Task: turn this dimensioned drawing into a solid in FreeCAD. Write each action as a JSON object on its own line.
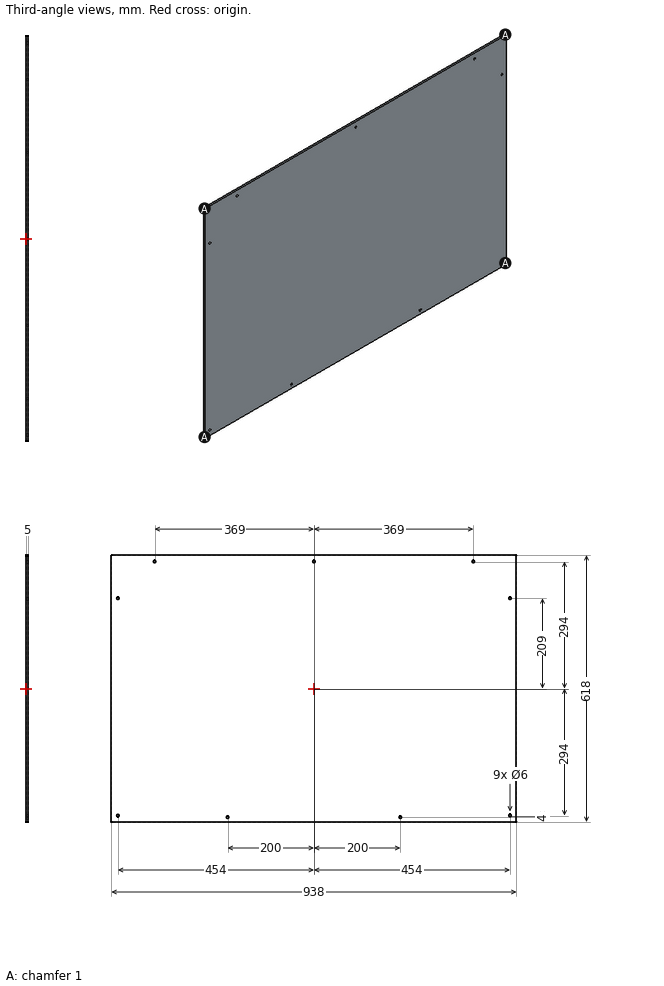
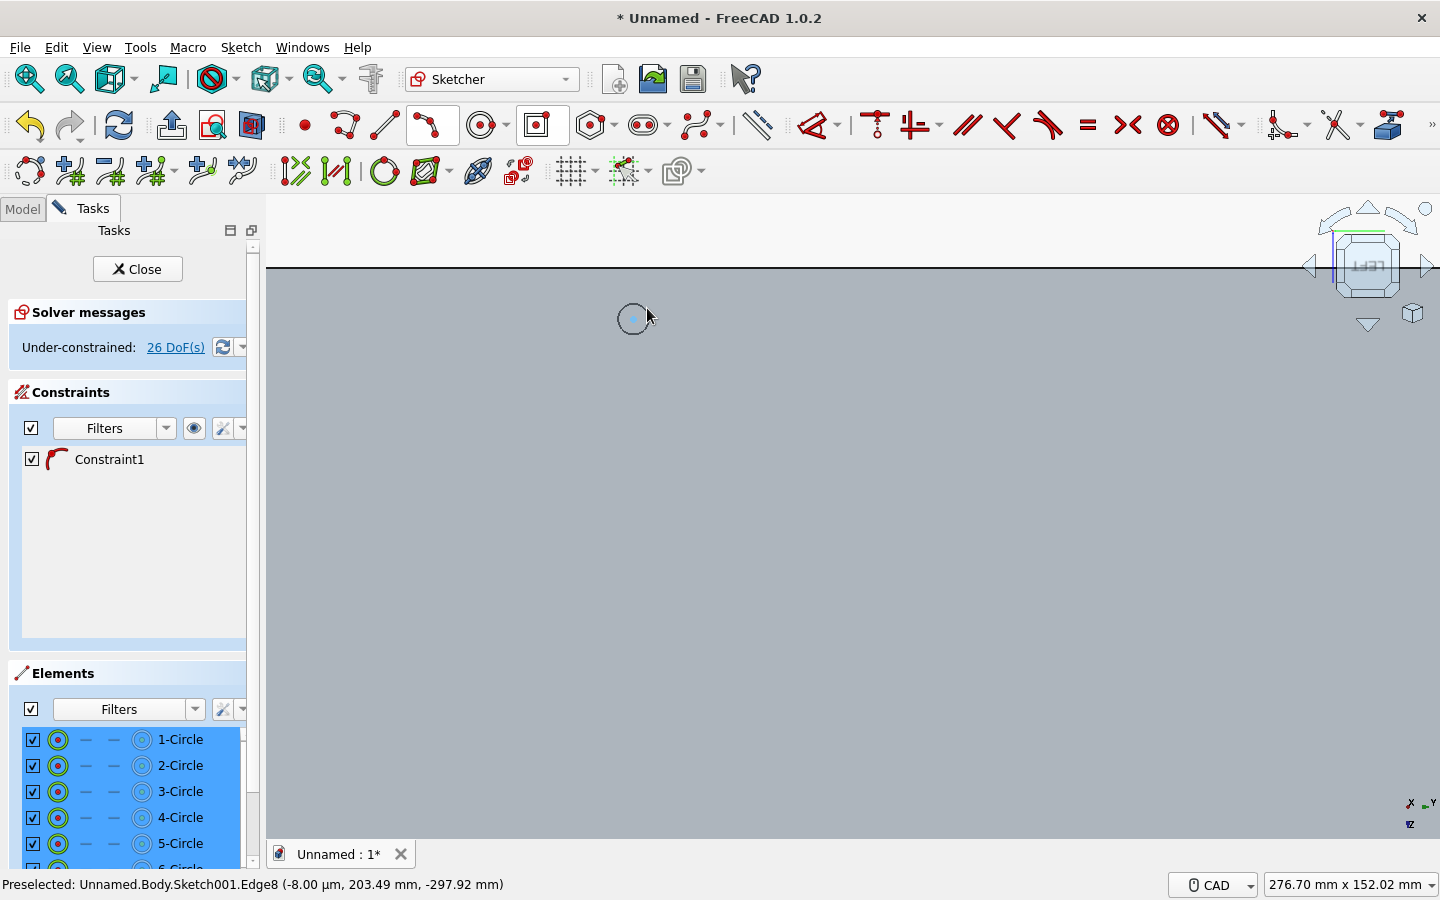
{"action": "left_click", "coordinate": [644, 308]}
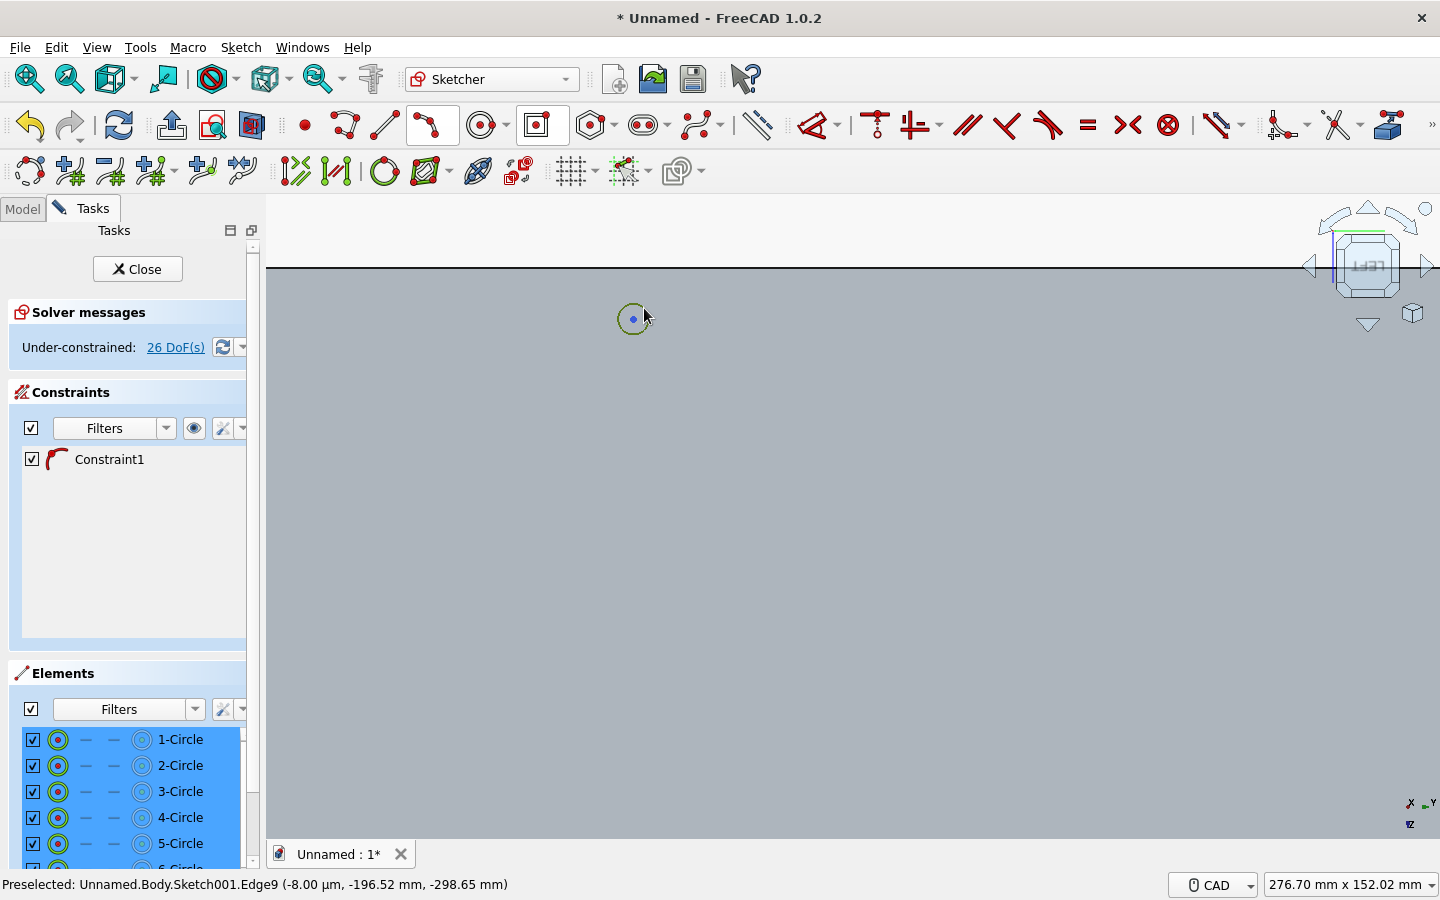
{"action": "left_click", "coordinate": [1088, 126]}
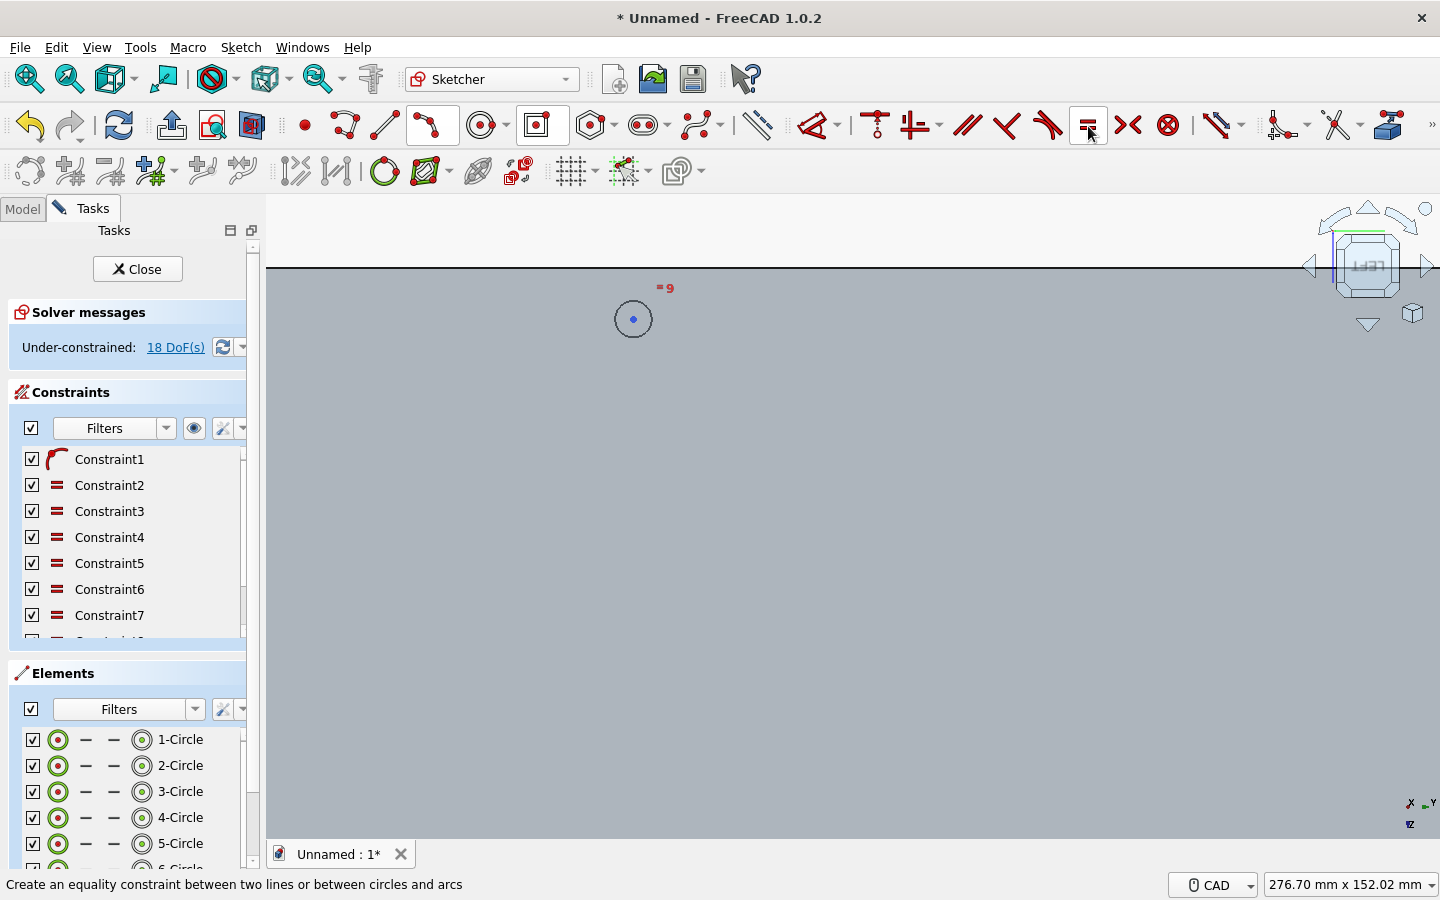
{"action": "scroll", "coordinate": [647, 308], "scroll_direction": "down", "scroll_amount": 9}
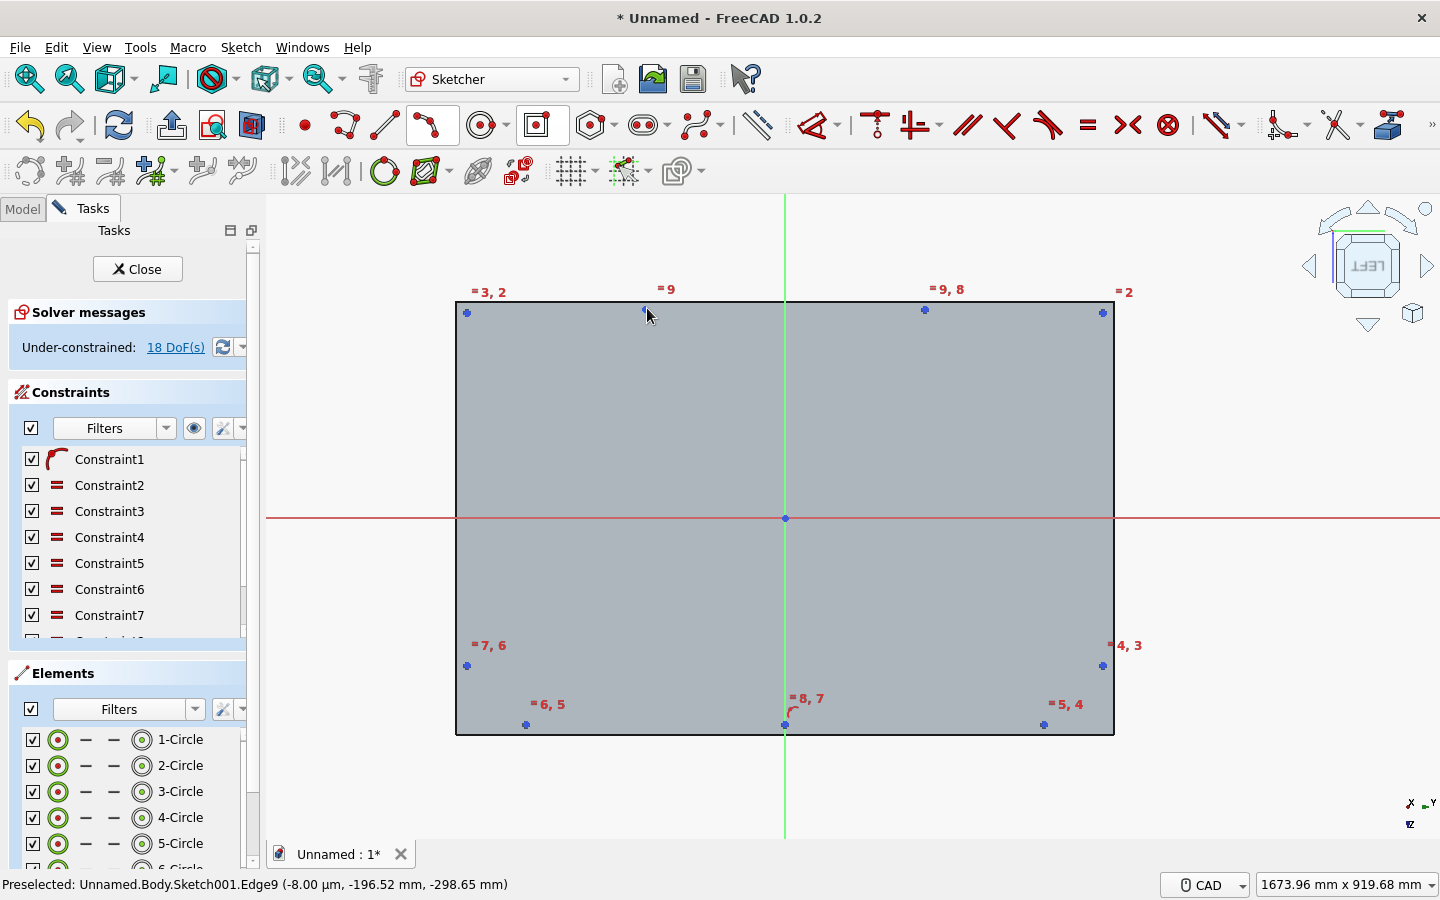
{"action": "left_click", "coordinate": [1103, 313]}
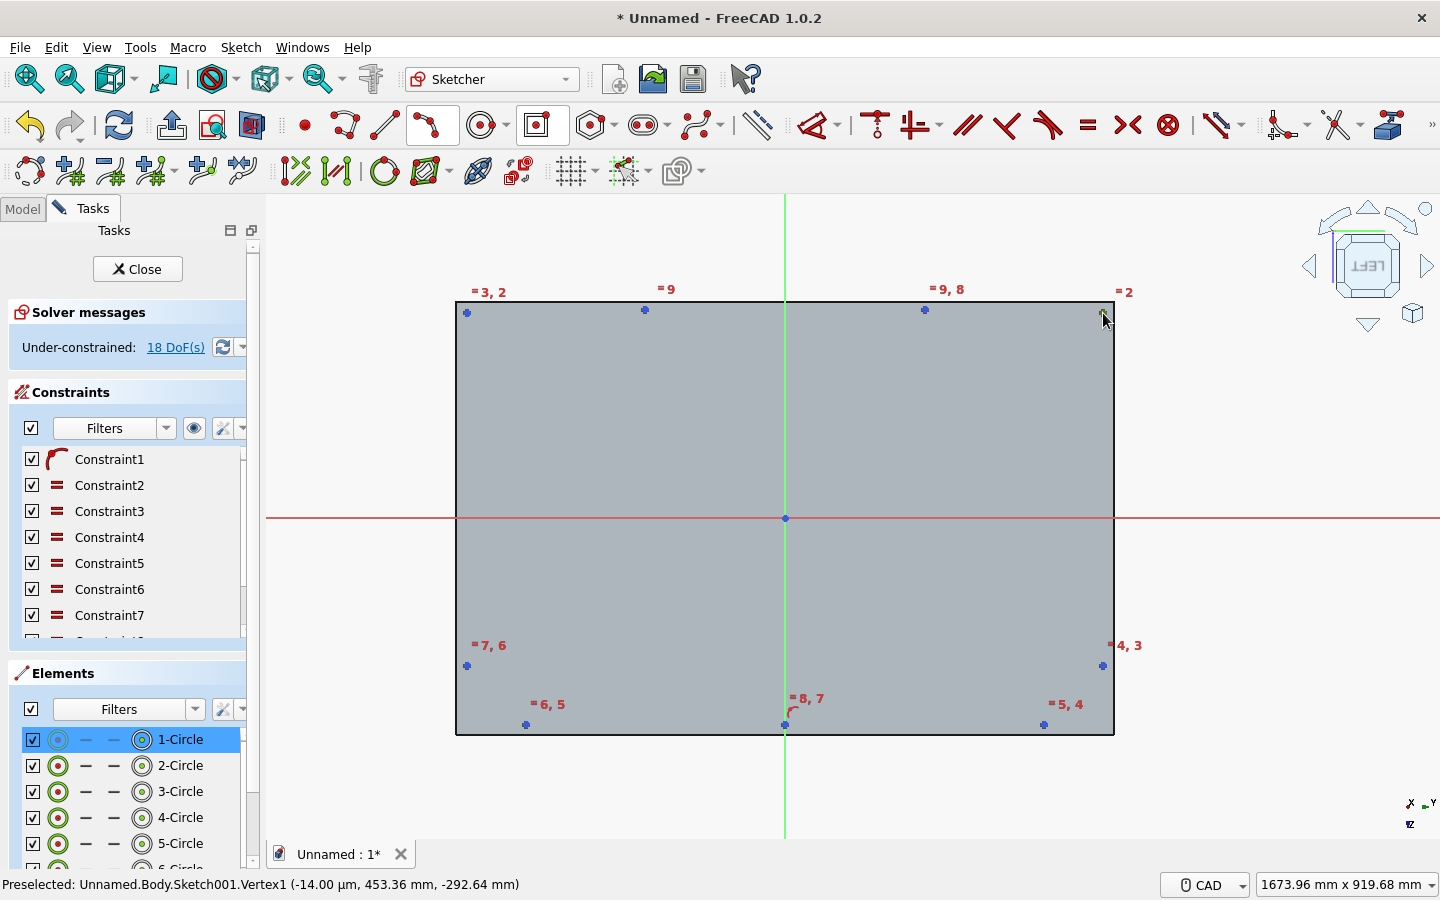
{"action": "left_click", "coordinate": [467, 313]}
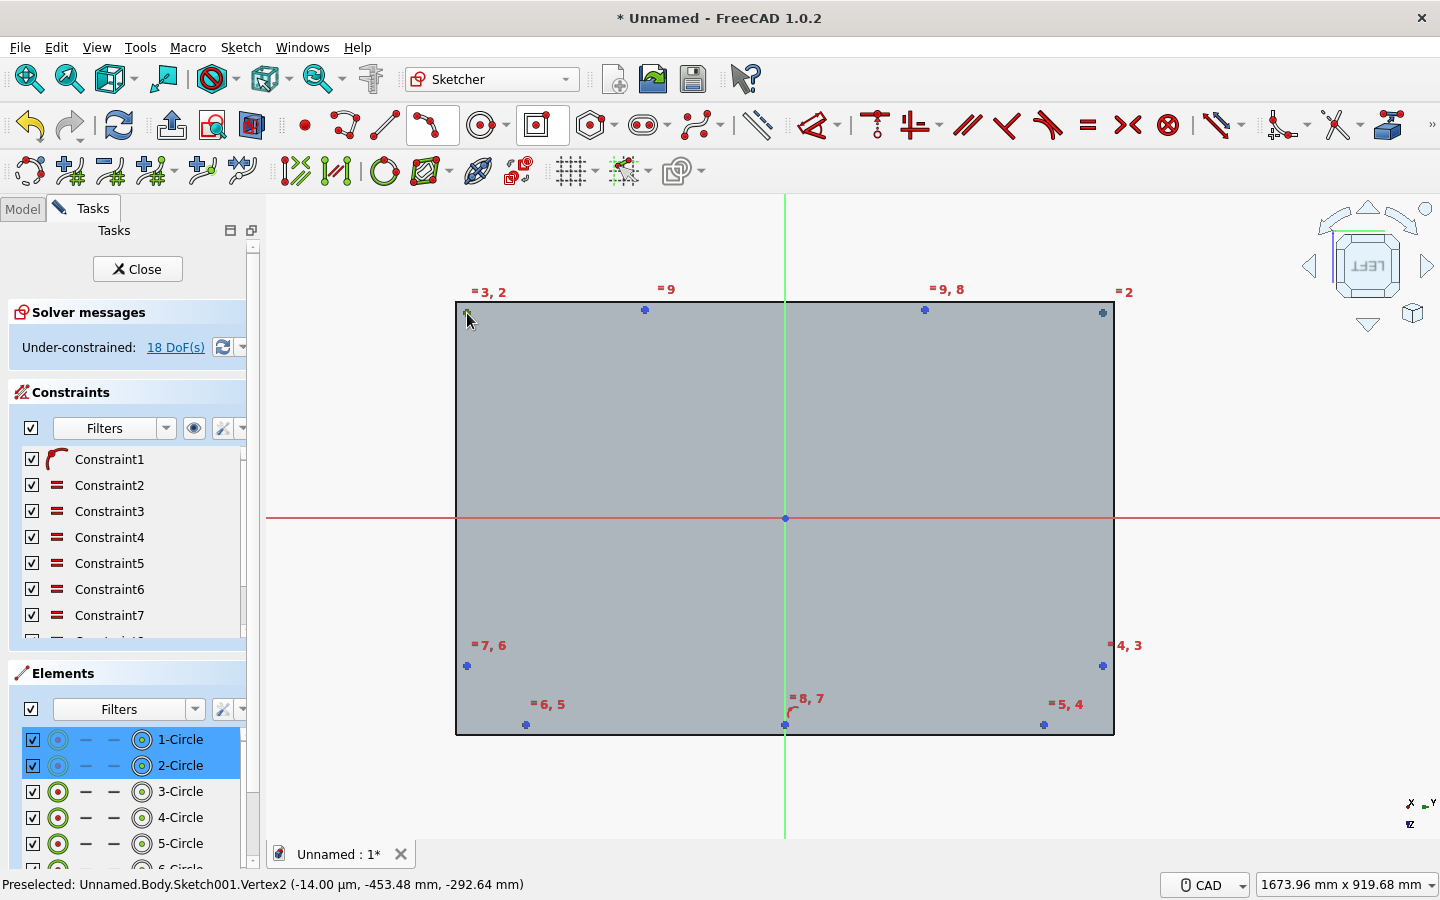
{"action": "key", "text": "h"}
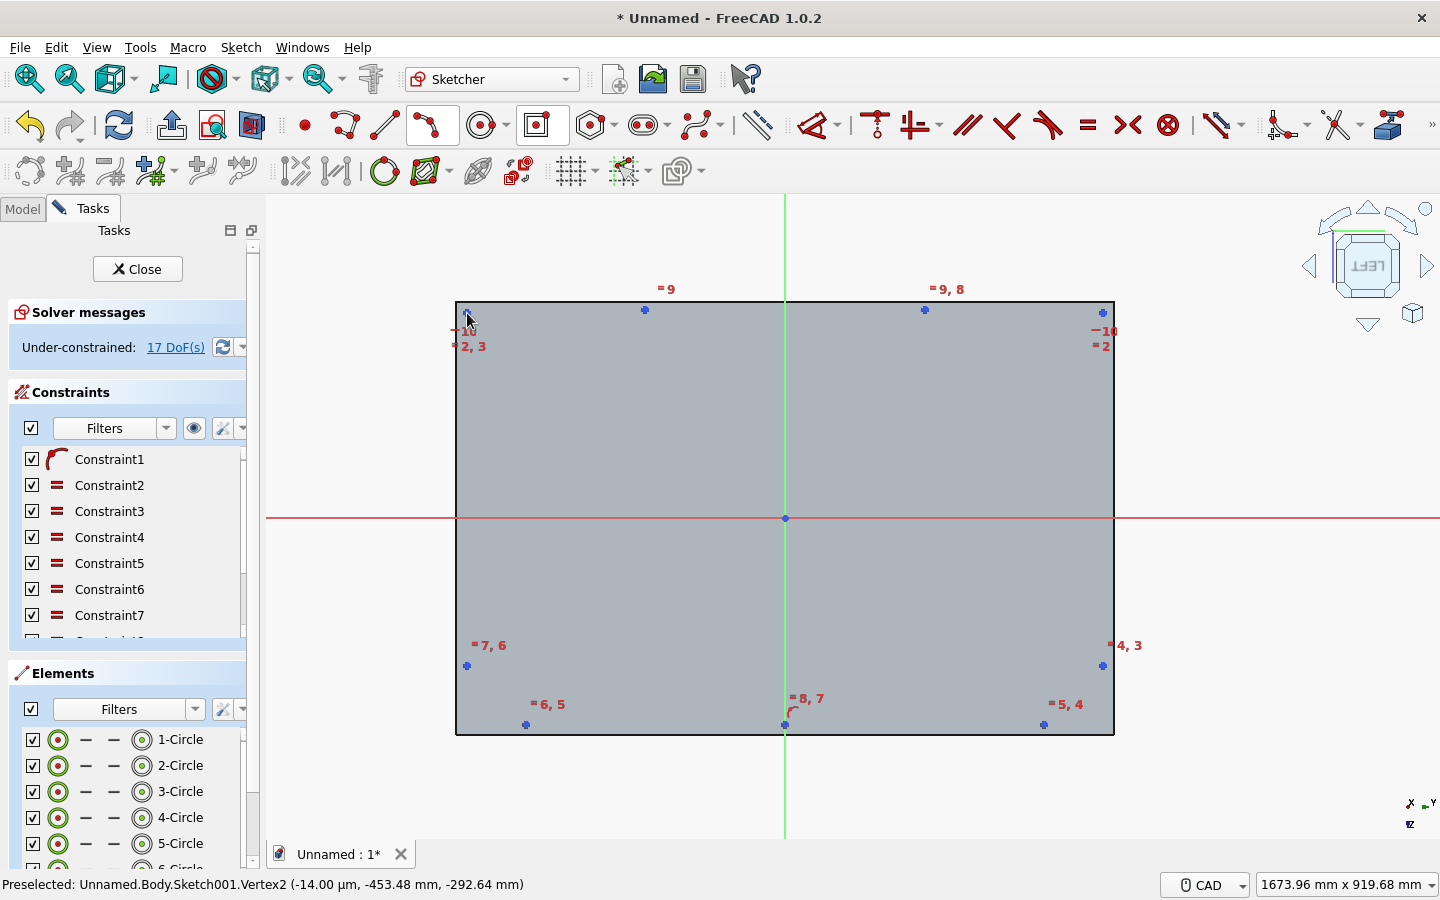
{"action": "left_click", "coordinate": [1103, 313]}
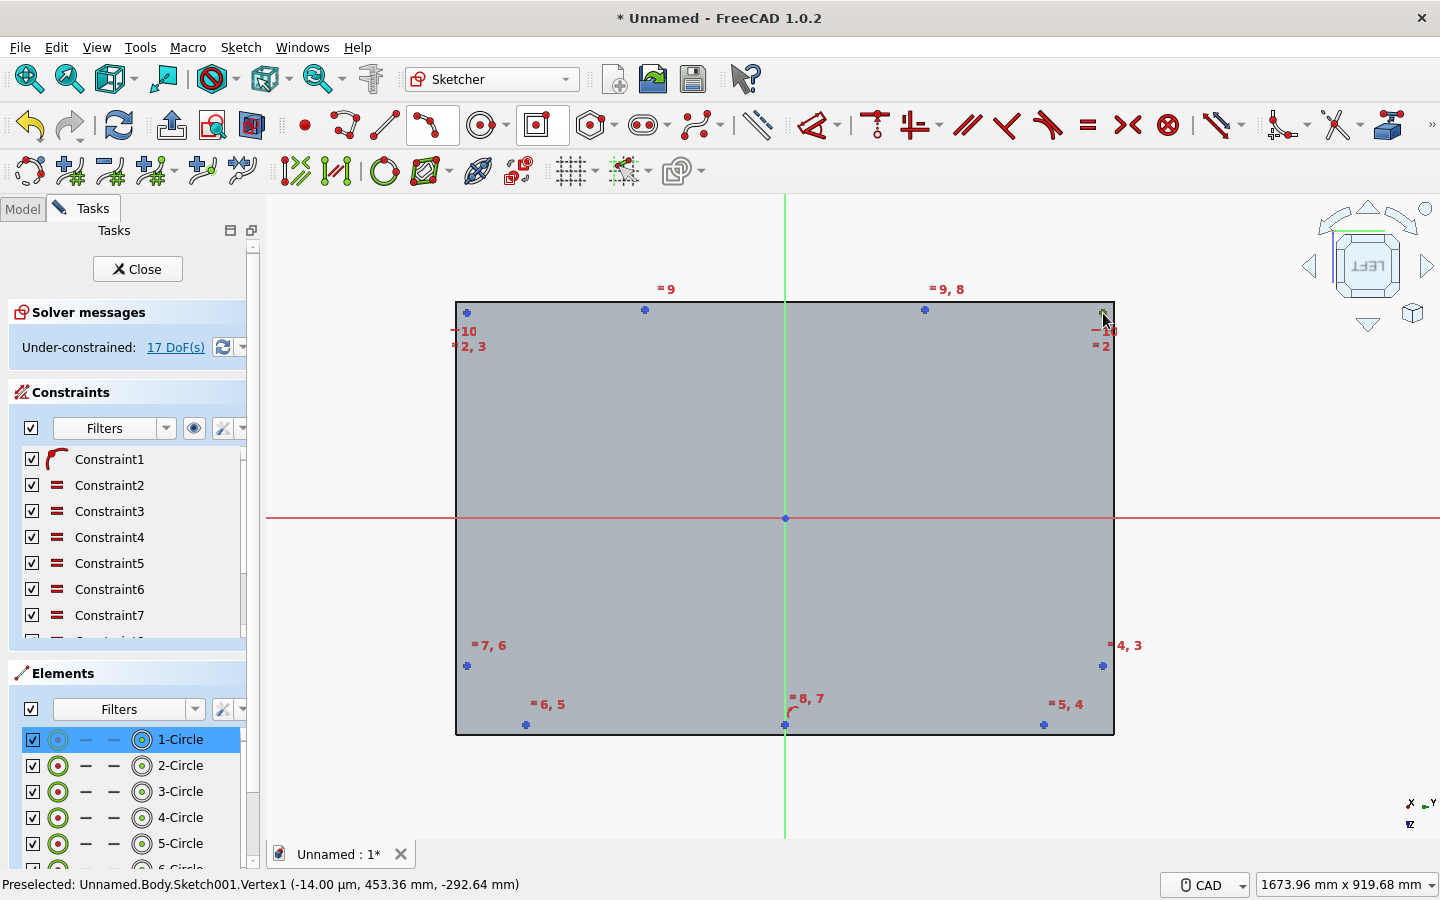
{"action": "left_click", "coordinate": [1103, 666]}